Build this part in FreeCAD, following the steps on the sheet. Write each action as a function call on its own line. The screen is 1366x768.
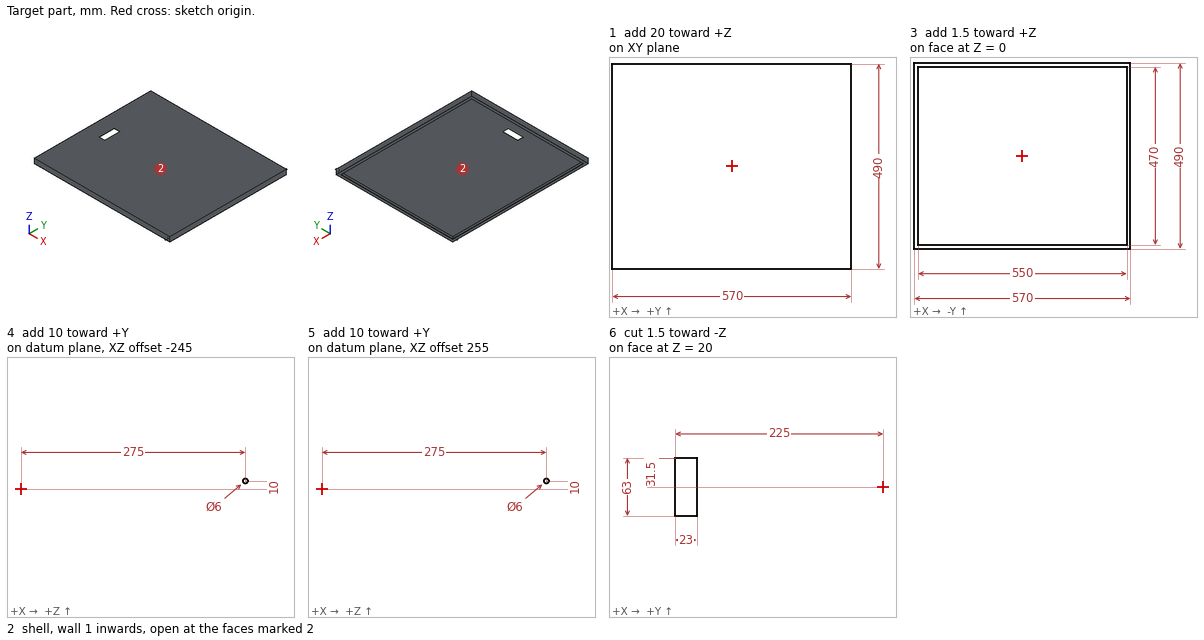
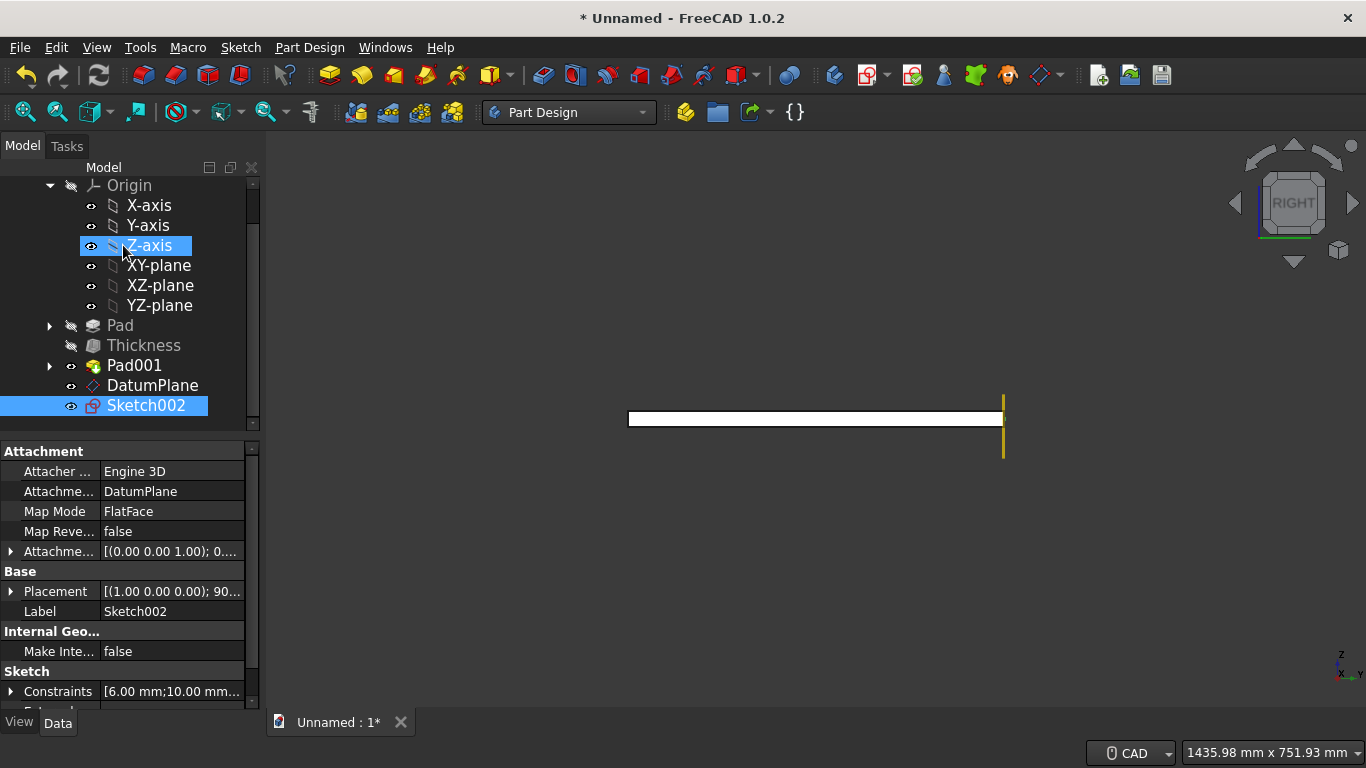
click(330, 76)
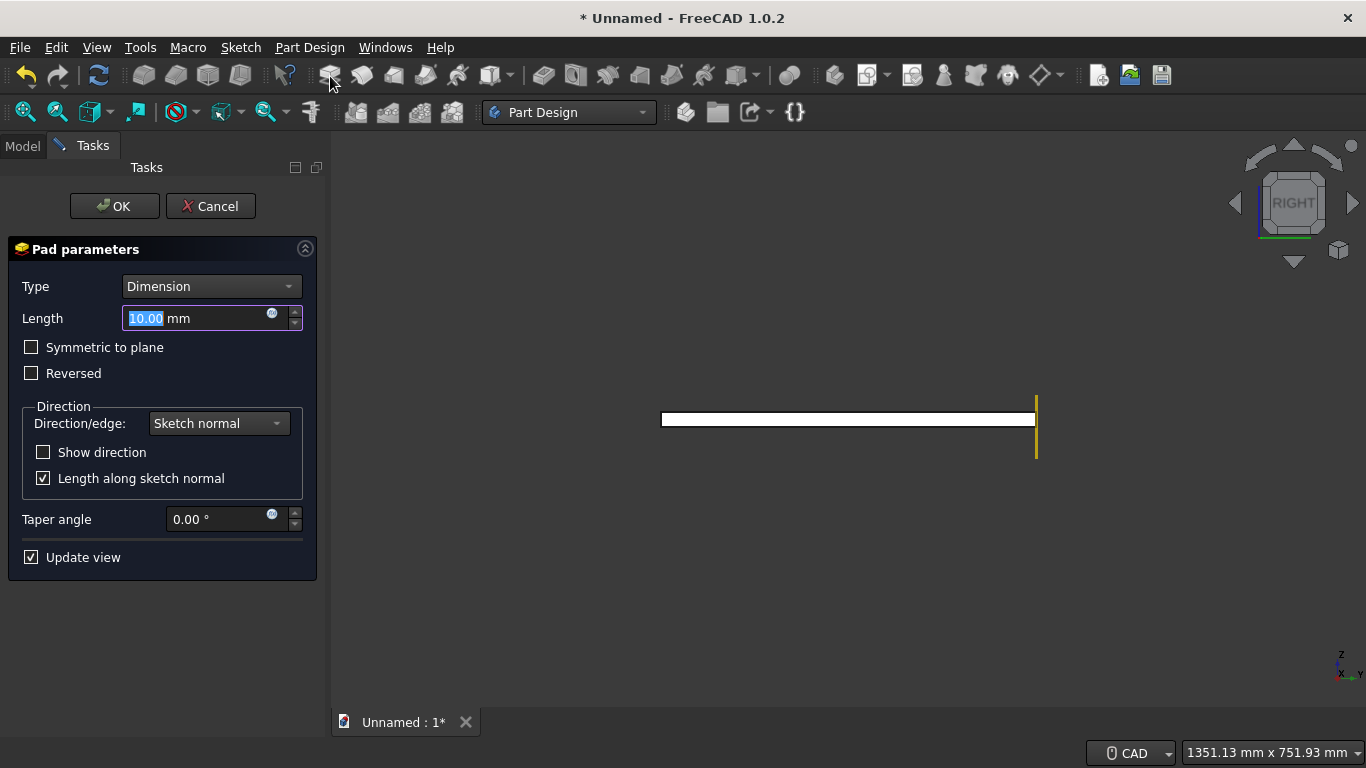
text(10)
key(Tab)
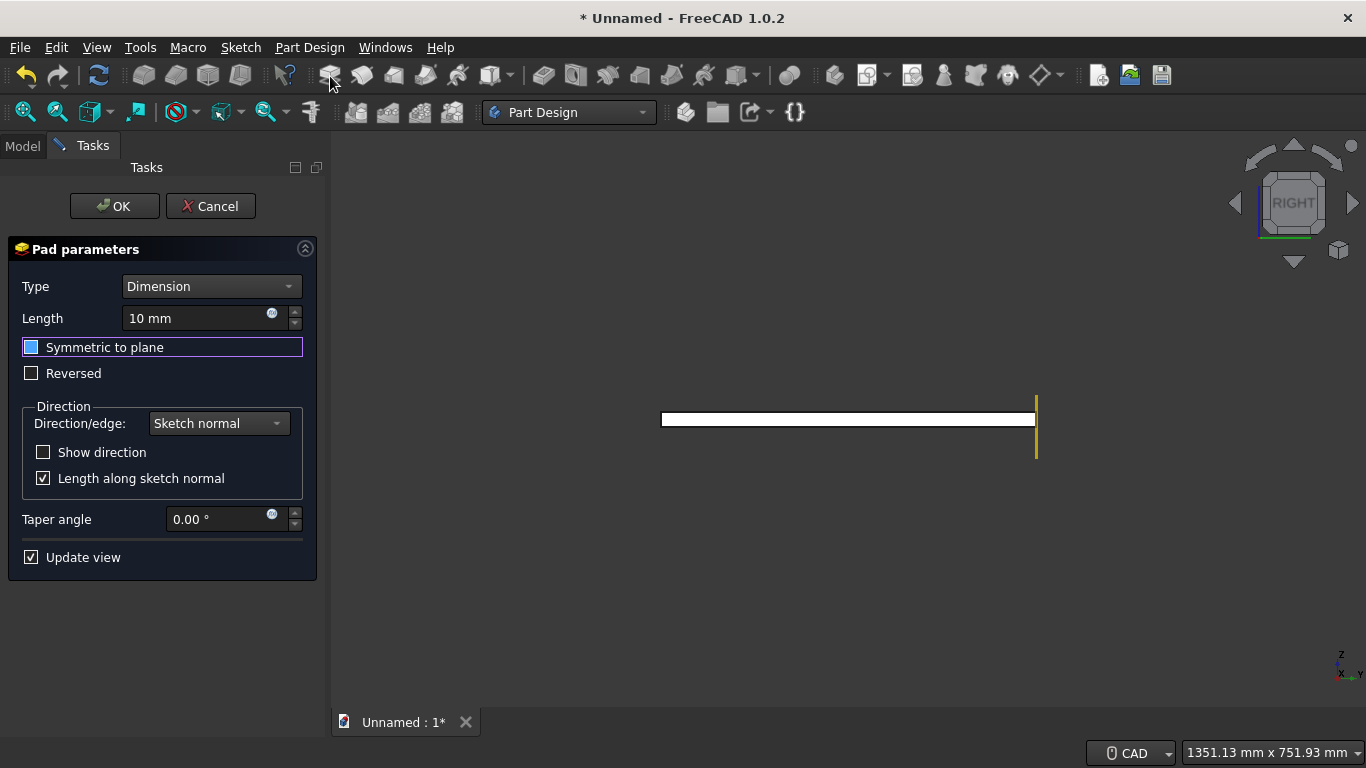
click(30, 373)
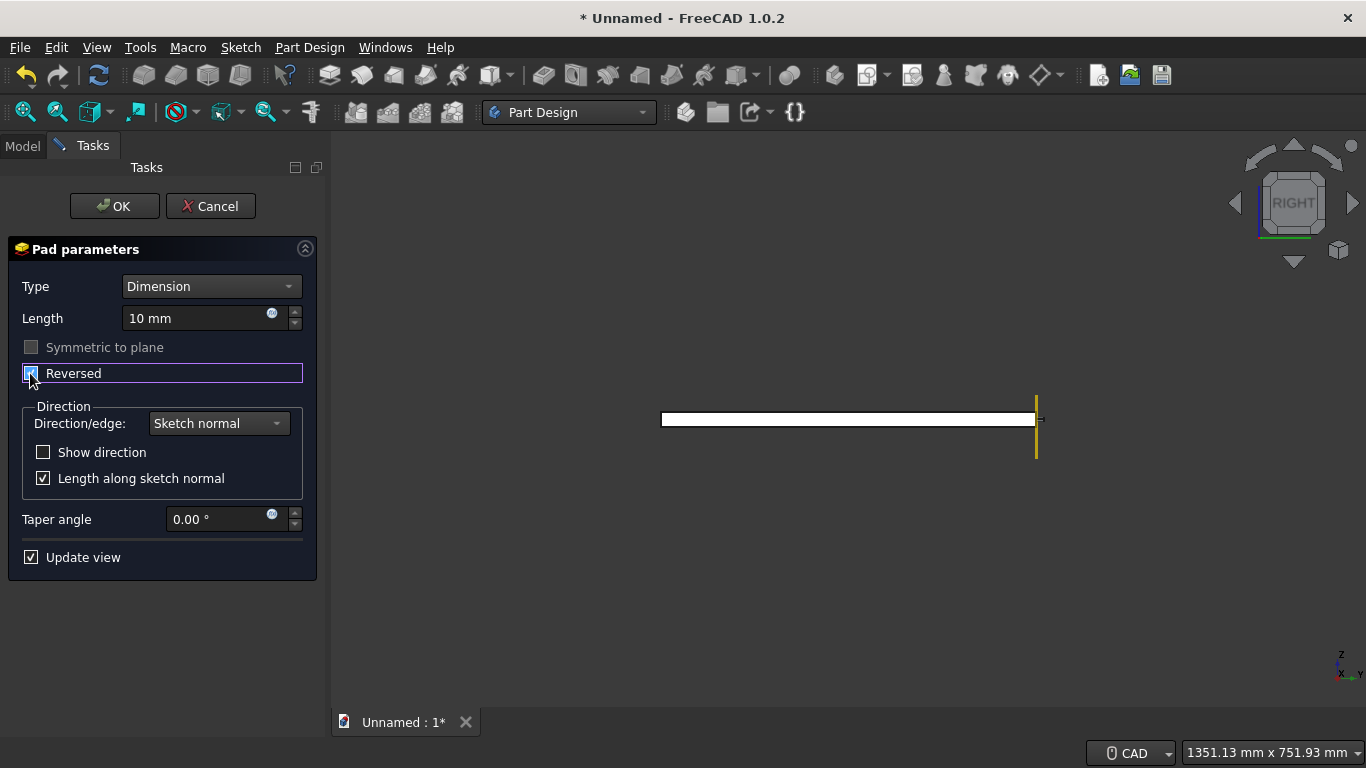
click(115, 206)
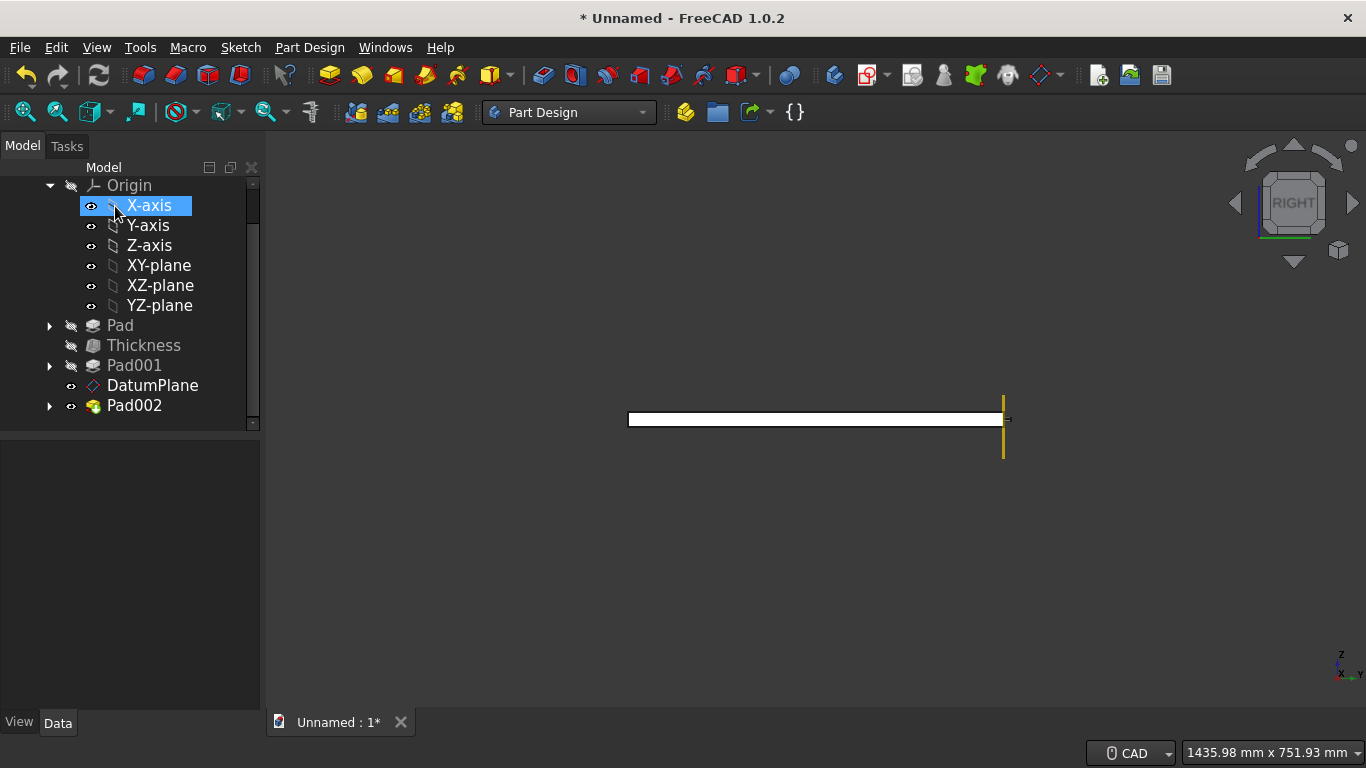
click(116, 386)
key(space)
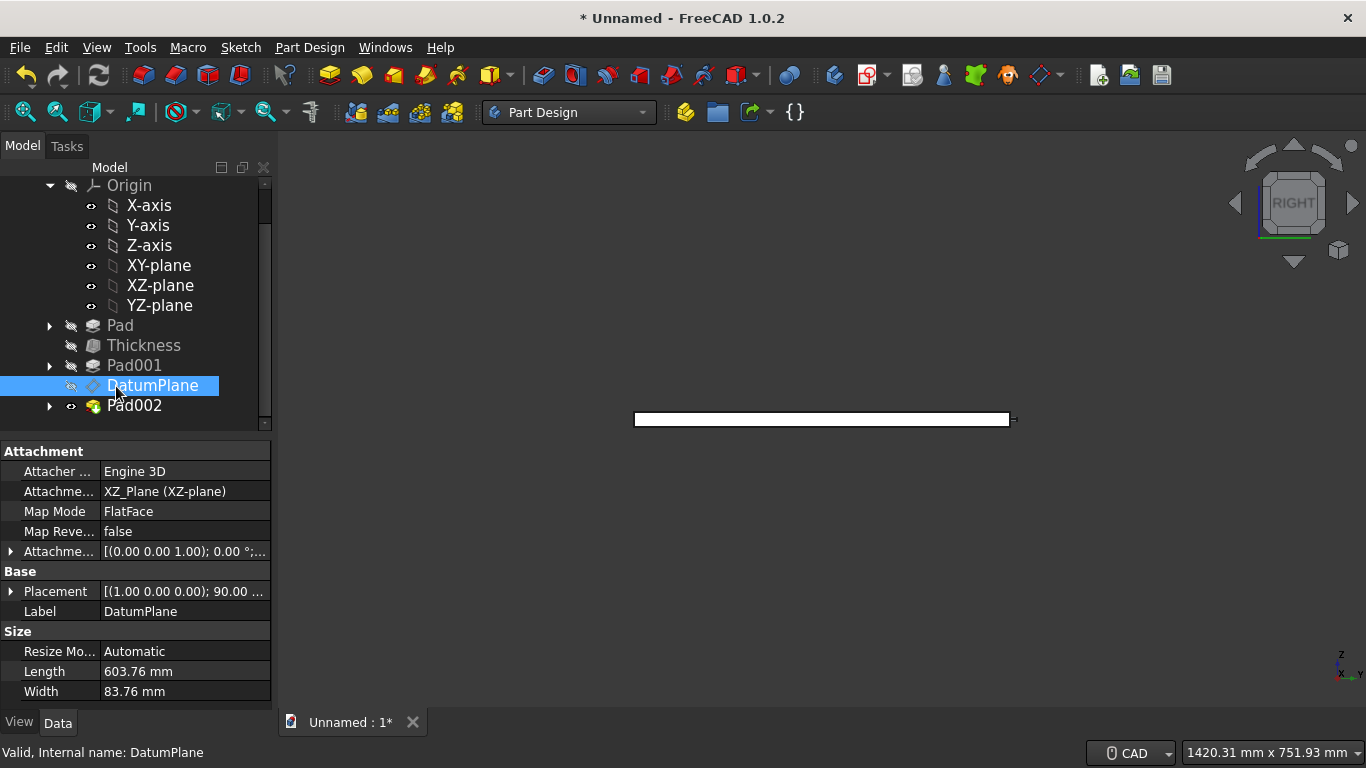
click(26, 112)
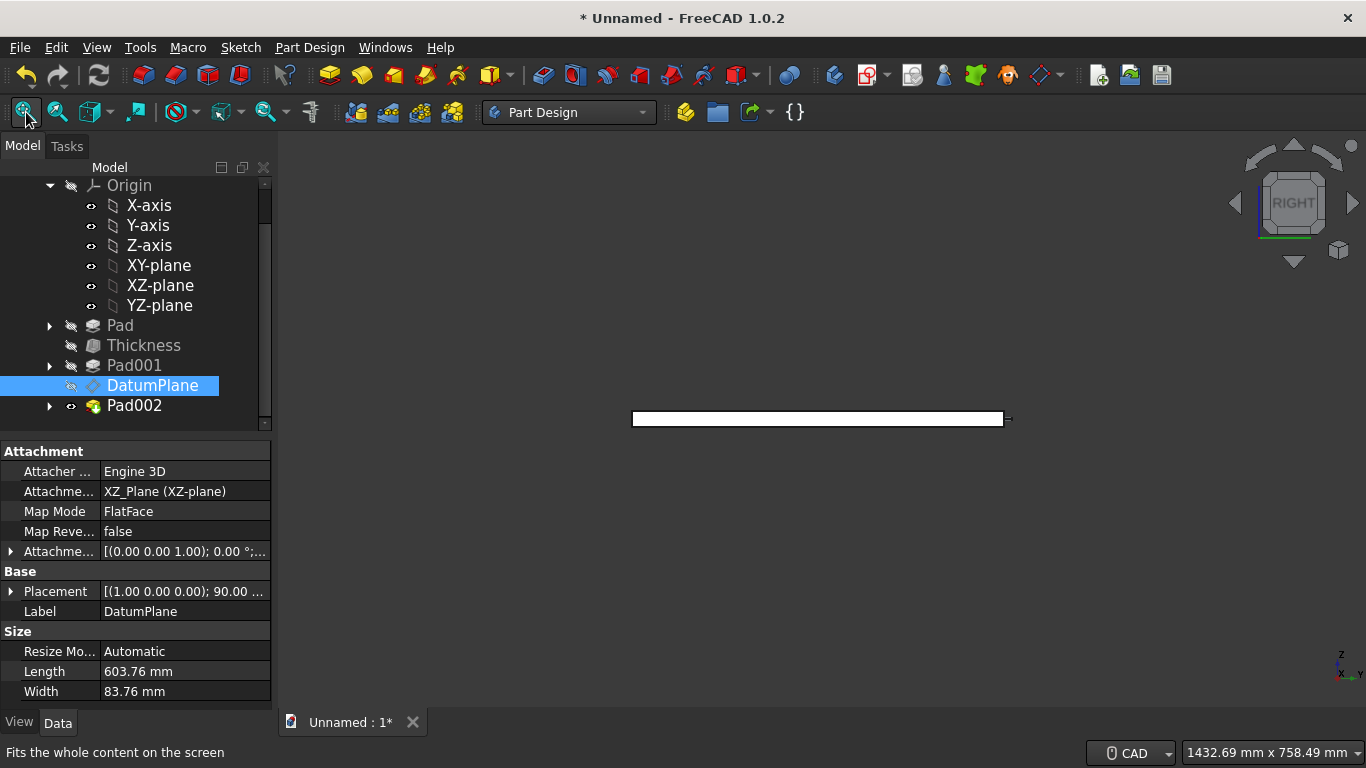
click(136, 286)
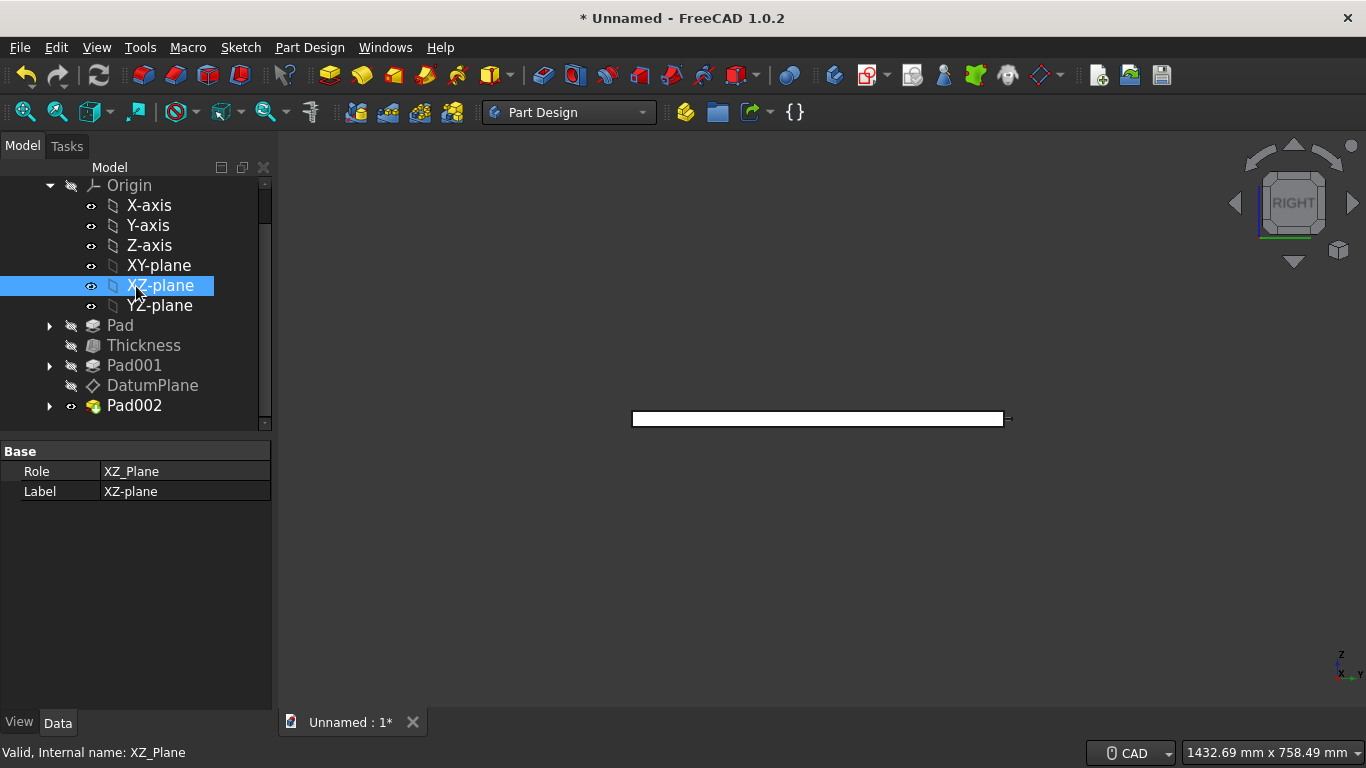
click(1040, 76)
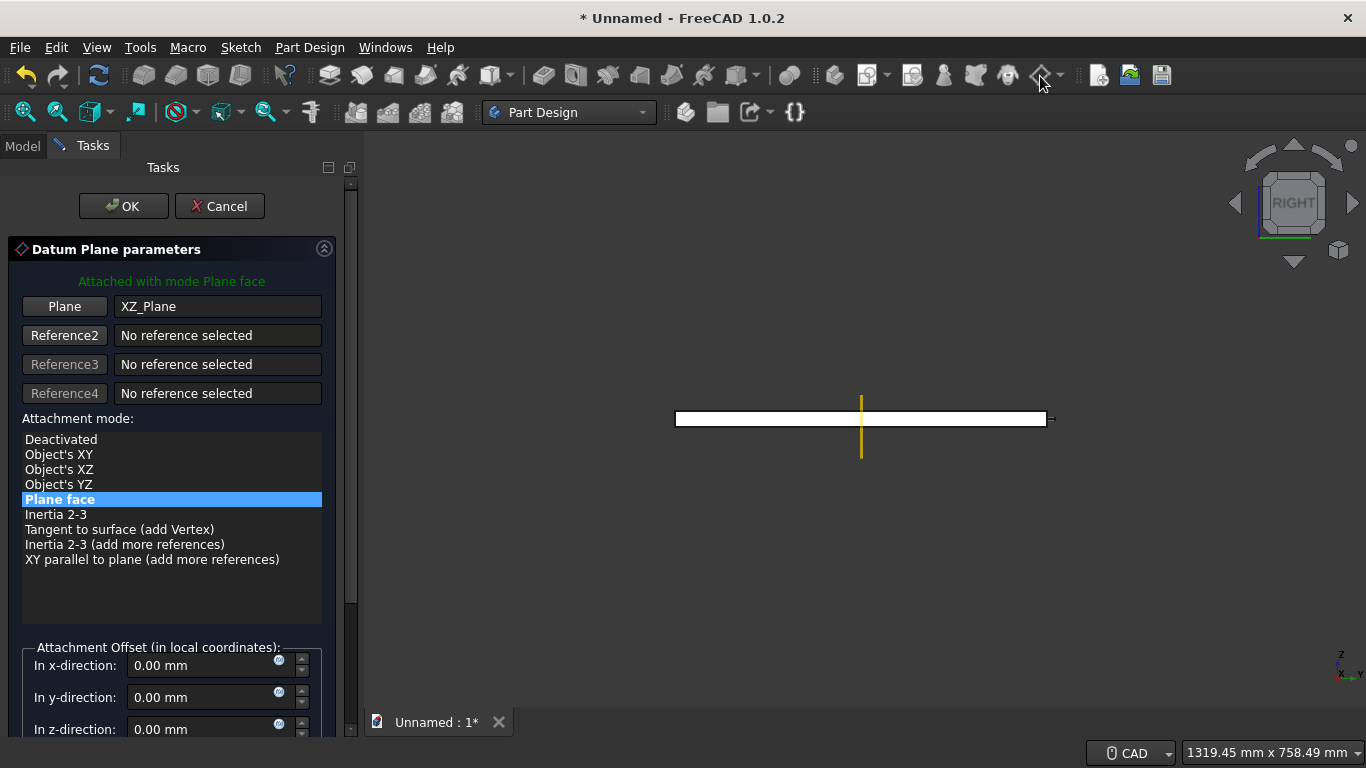
scroll(351, 456, down, 2)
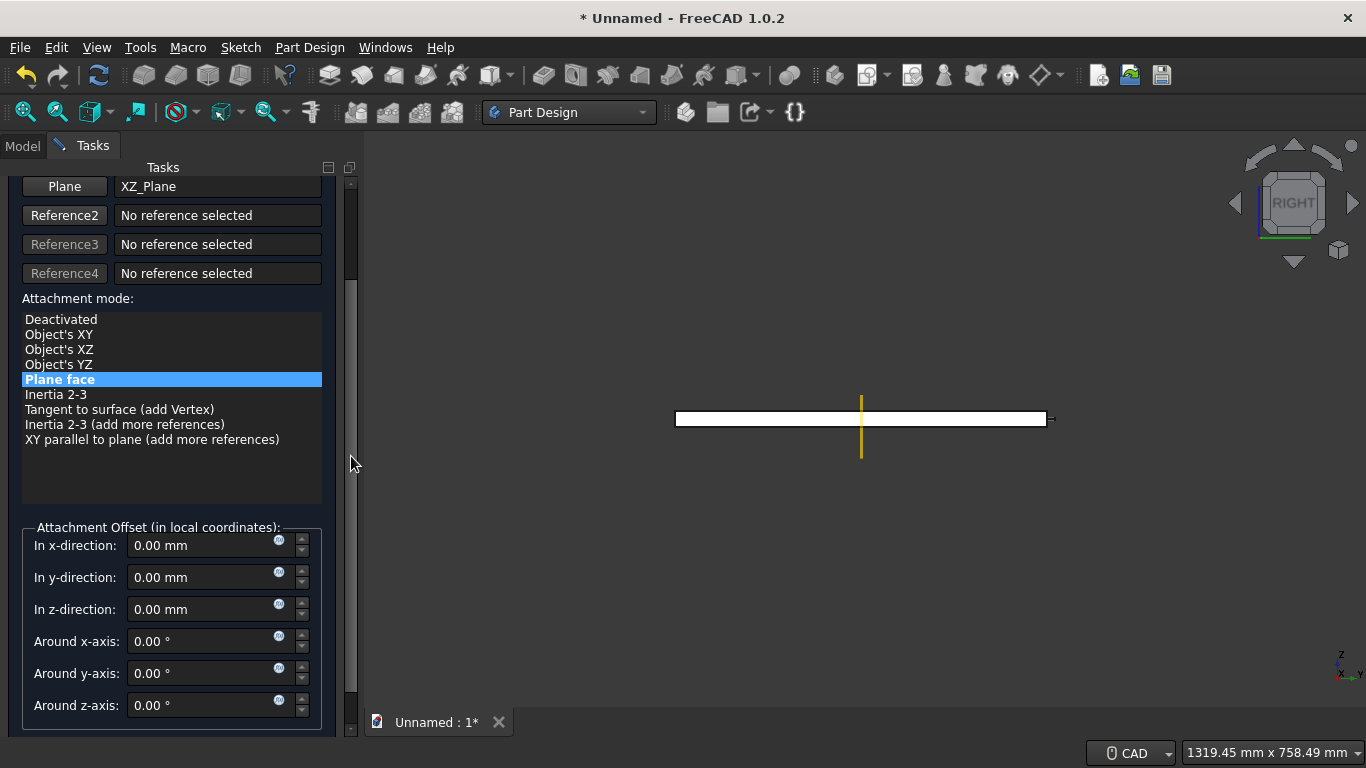
triple_click(210, 609)